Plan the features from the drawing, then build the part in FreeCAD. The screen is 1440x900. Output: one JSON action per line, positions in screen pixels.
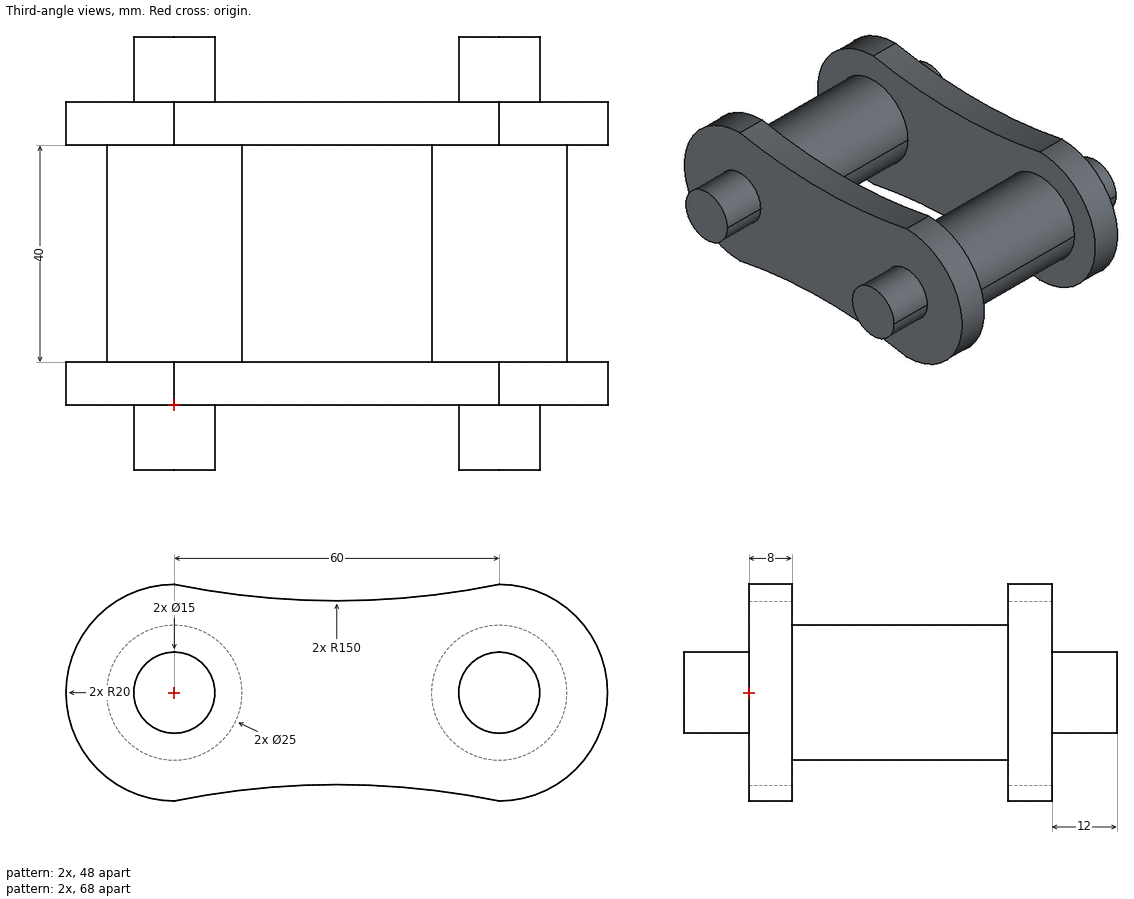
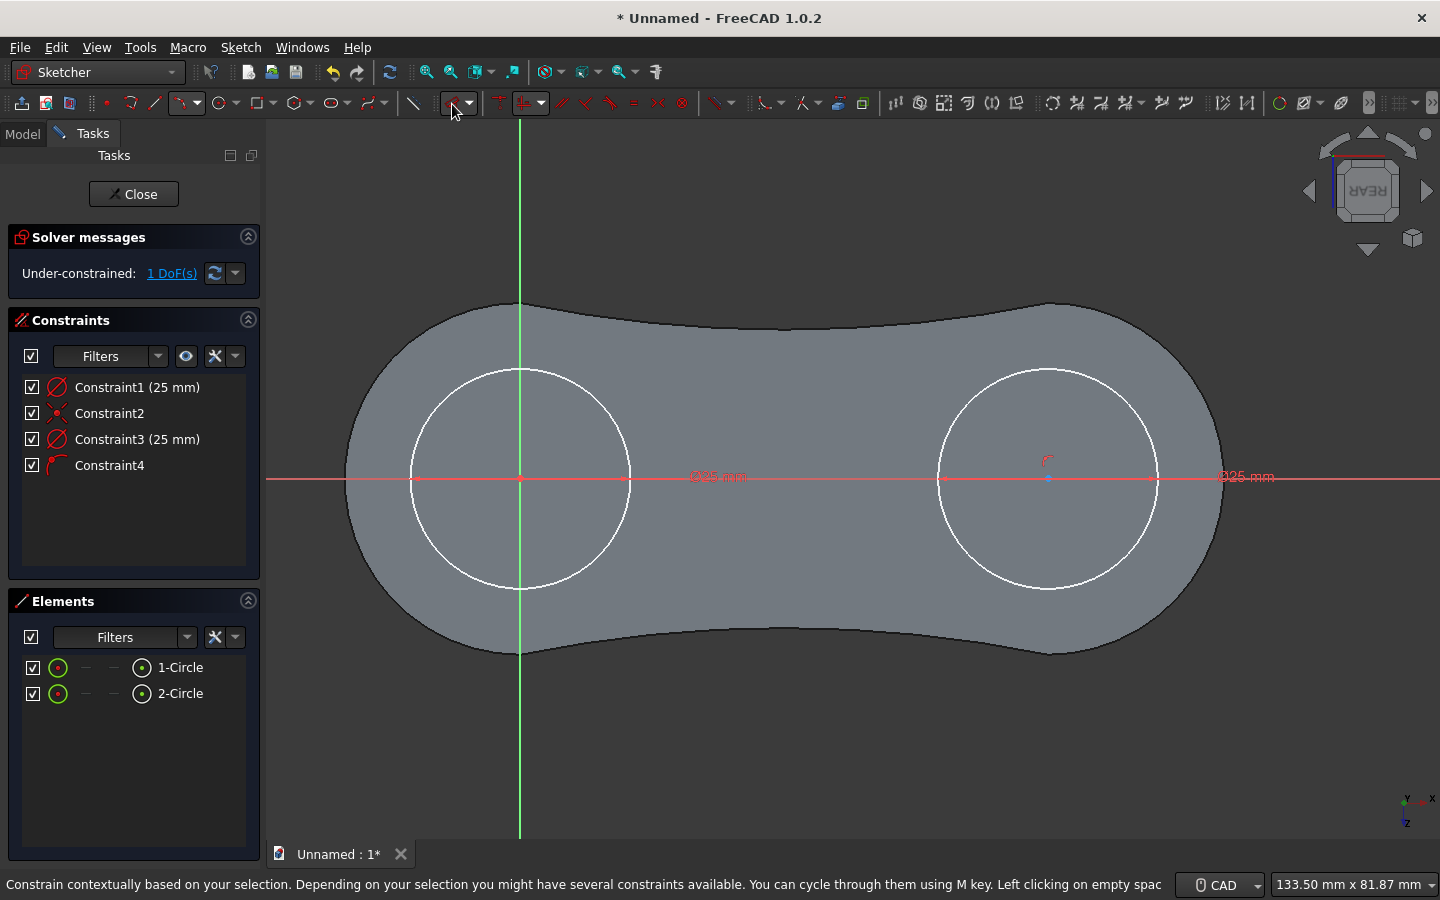
{"action": "left_click", "coordinate": [1048, 479]}
{"action": "left_click", "coordinate": [784, 513]}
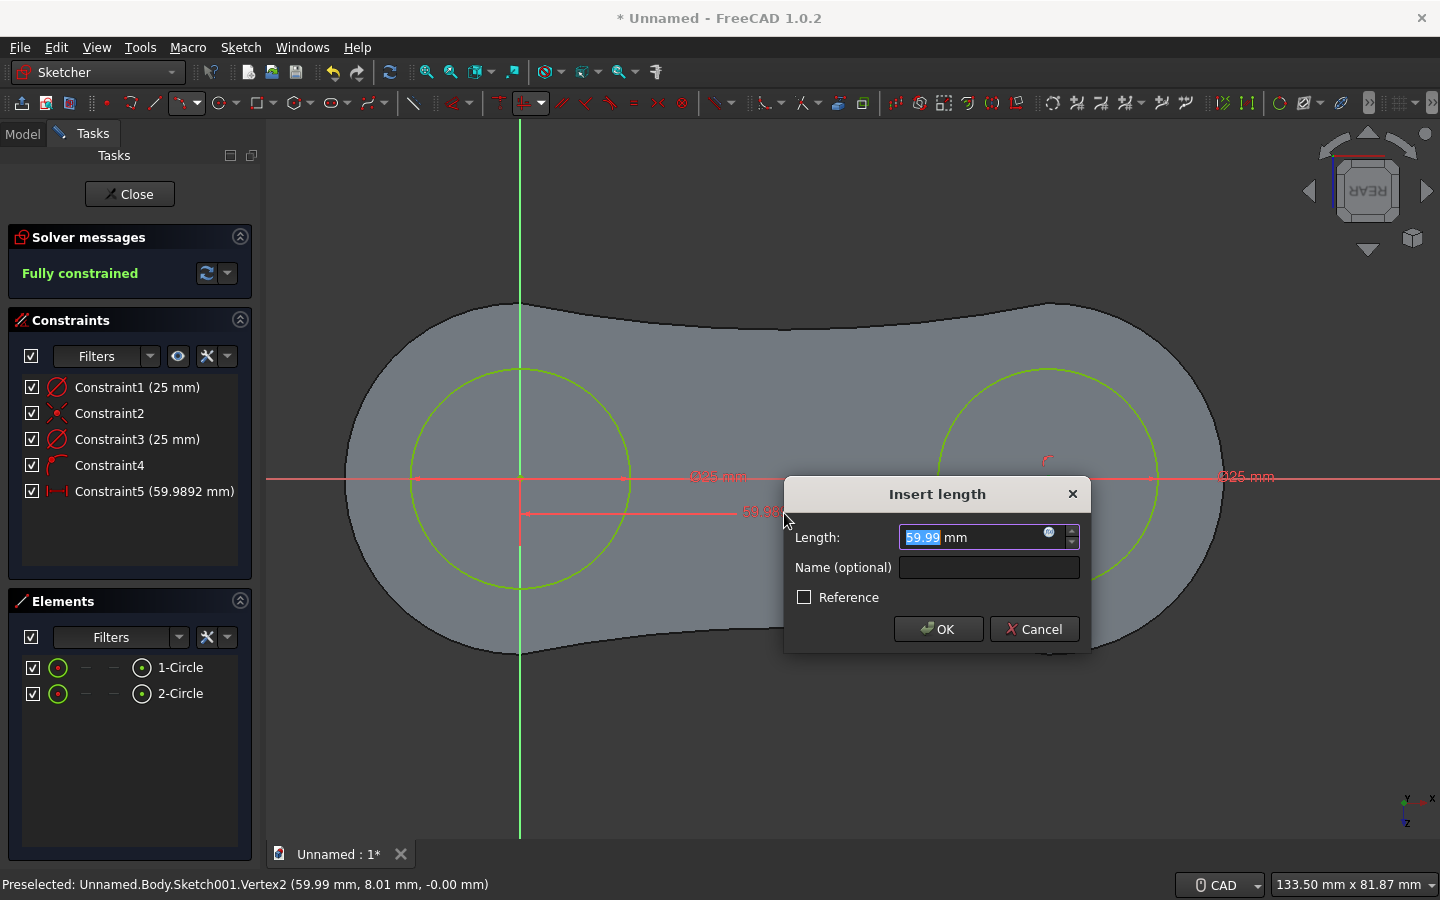
{"action": "type", "text": "60"}
{"action": "key", "text": "Return"}
{"action": "key", "text": "Escape"}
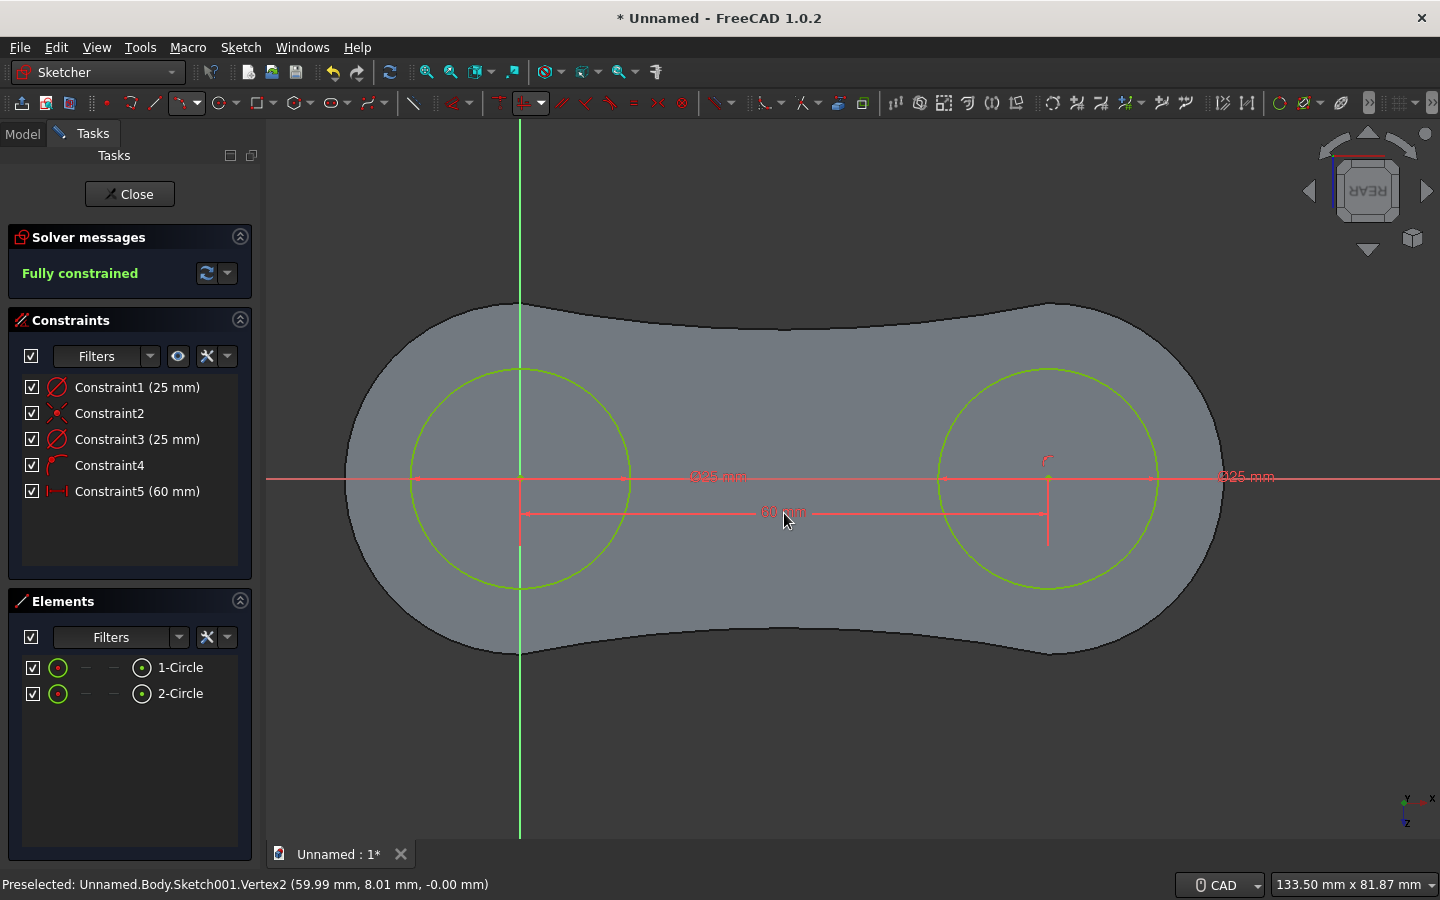
{"action": "left_click", "coordinate": [130, 194]}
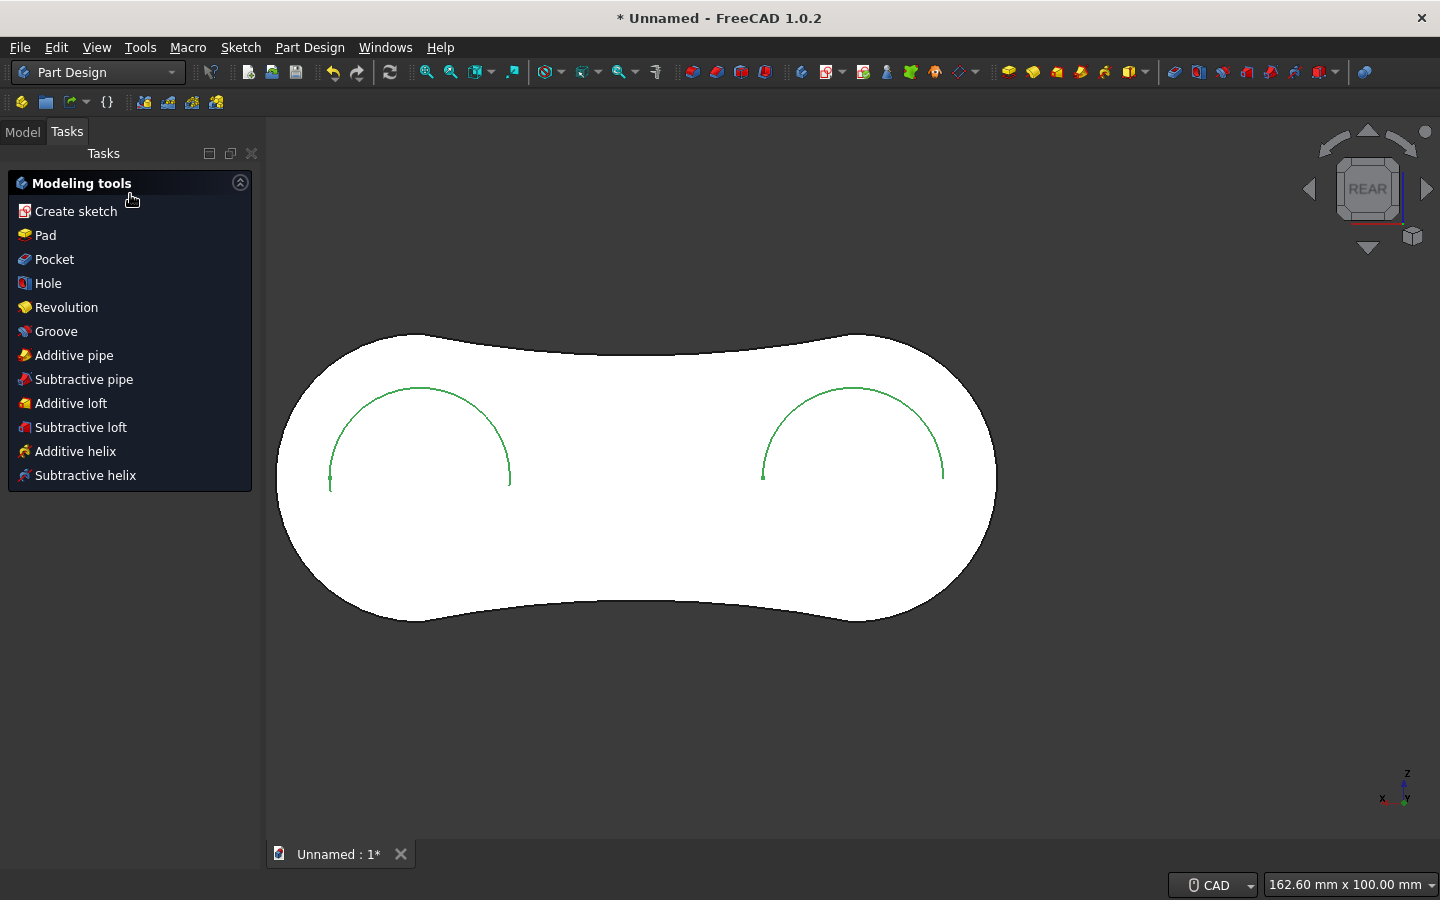
{"action": "left_click", "coordinate": [1010, 72]}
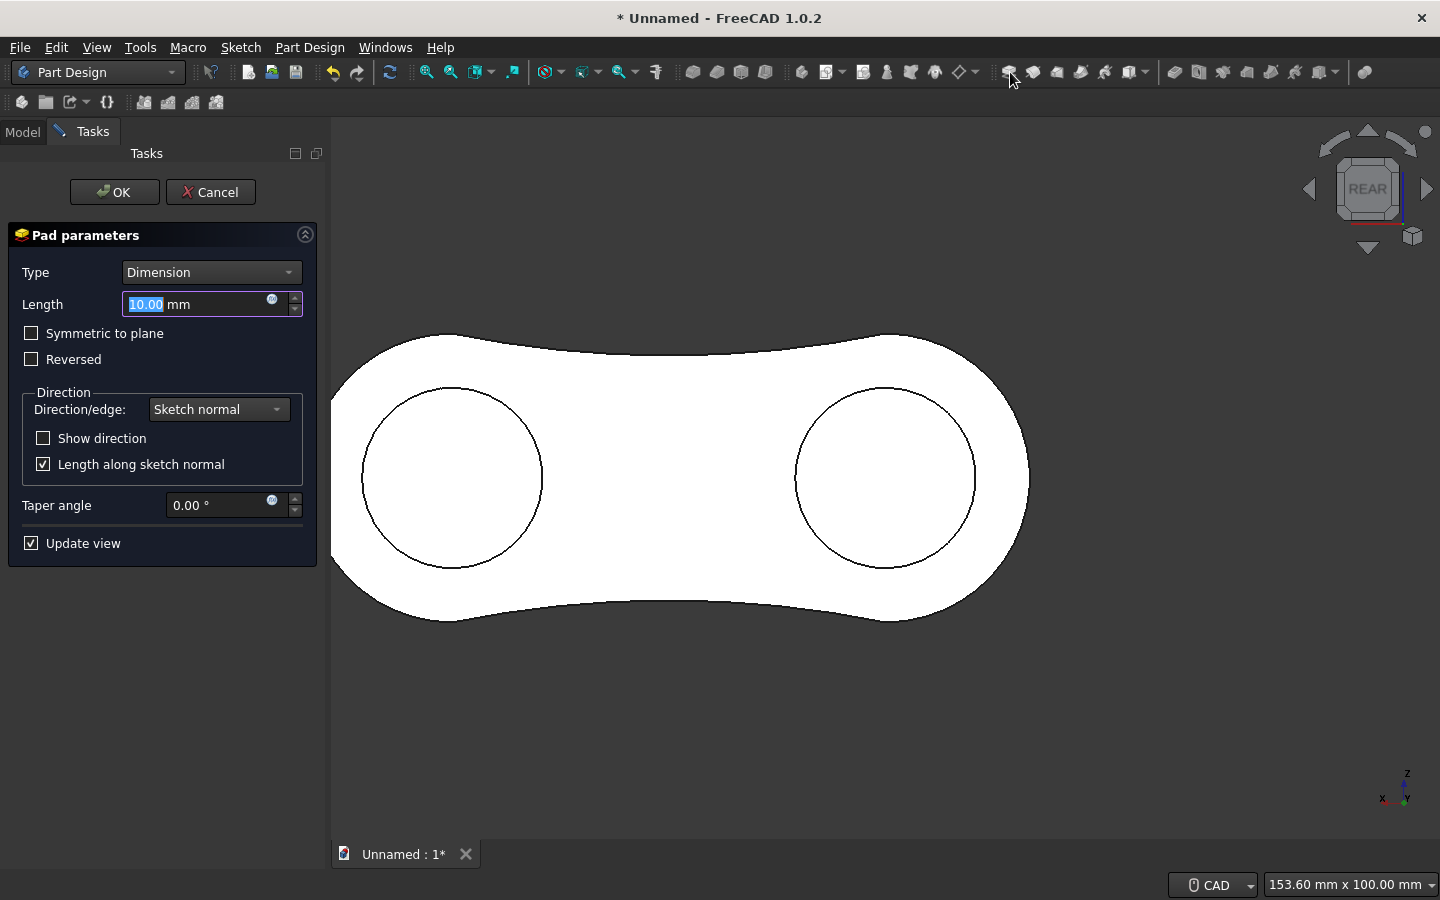
{"action": "type", "text": "40"}
{"action": "key", "text": "Tab"}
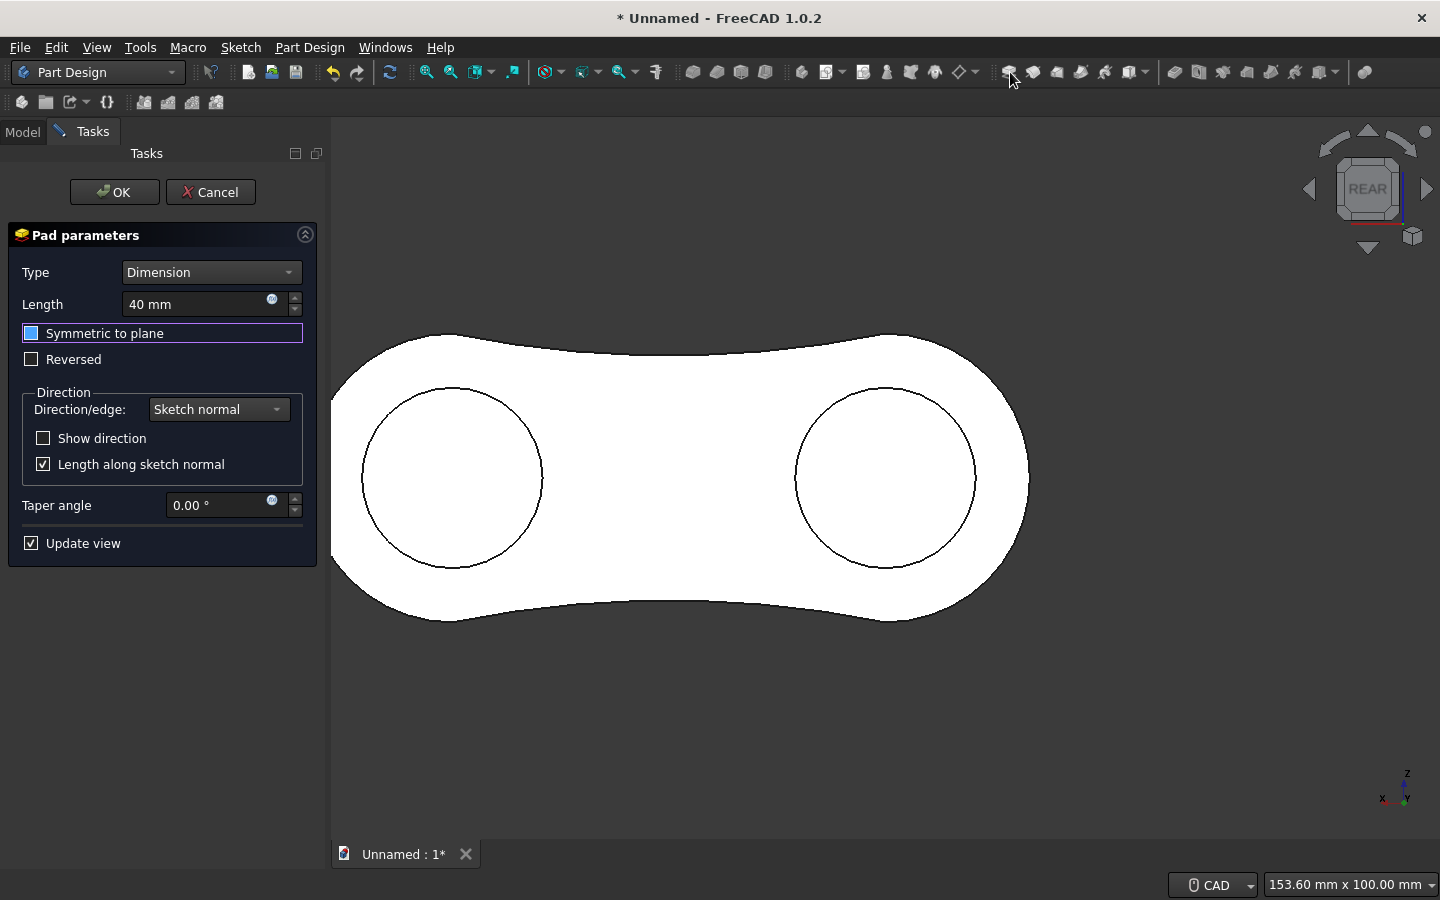
{"action": "left_click", "coordinate": [115, 192]}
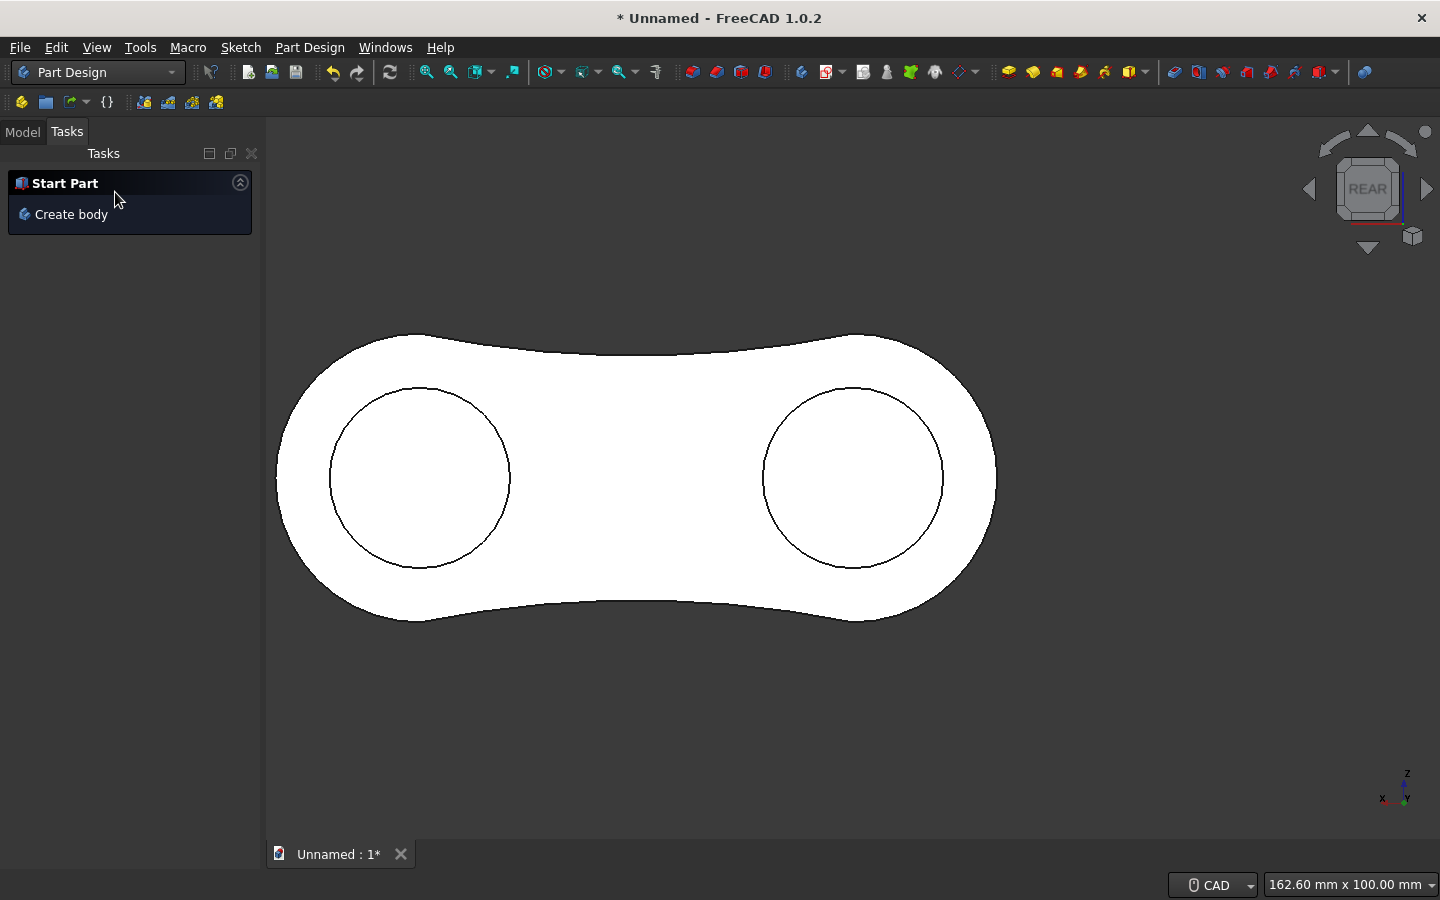
{"action": "left_click", "coordinate": [23, 131]}